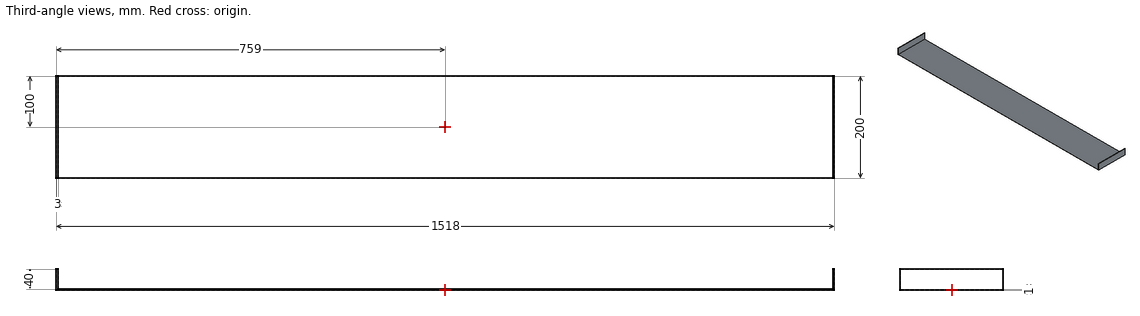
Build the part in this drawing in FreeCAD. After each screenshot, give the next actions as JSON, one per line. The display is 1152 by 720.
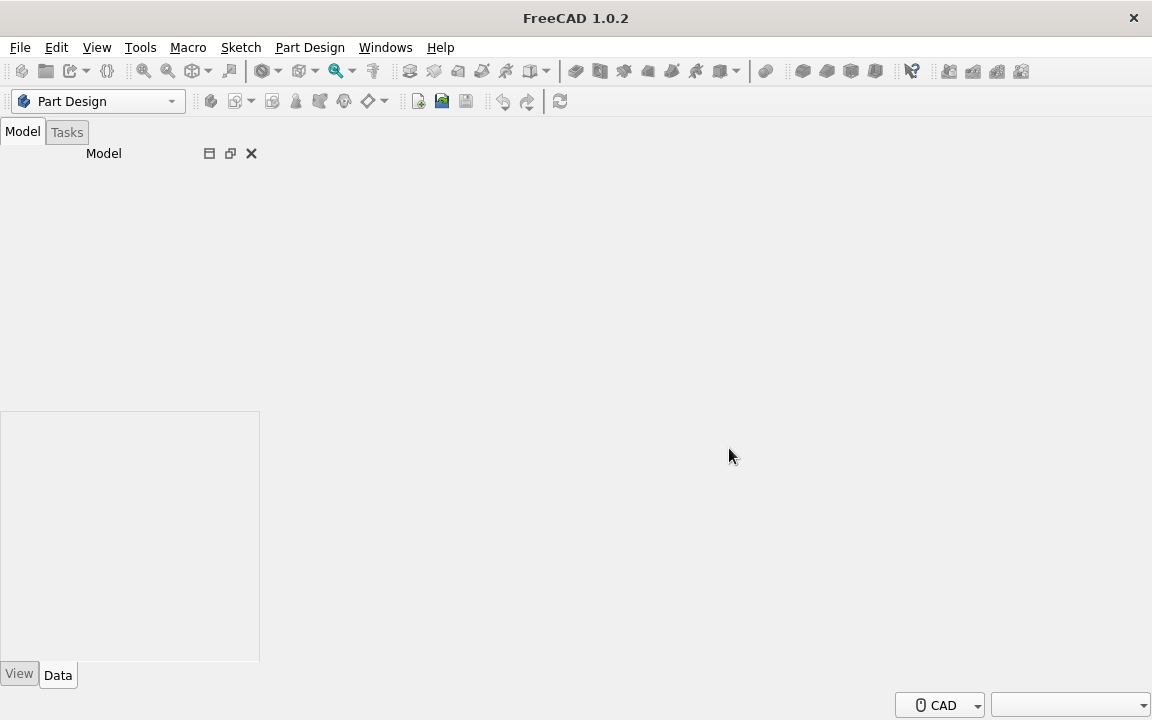
{"action": "left_click", "coordinate": [418, 102]}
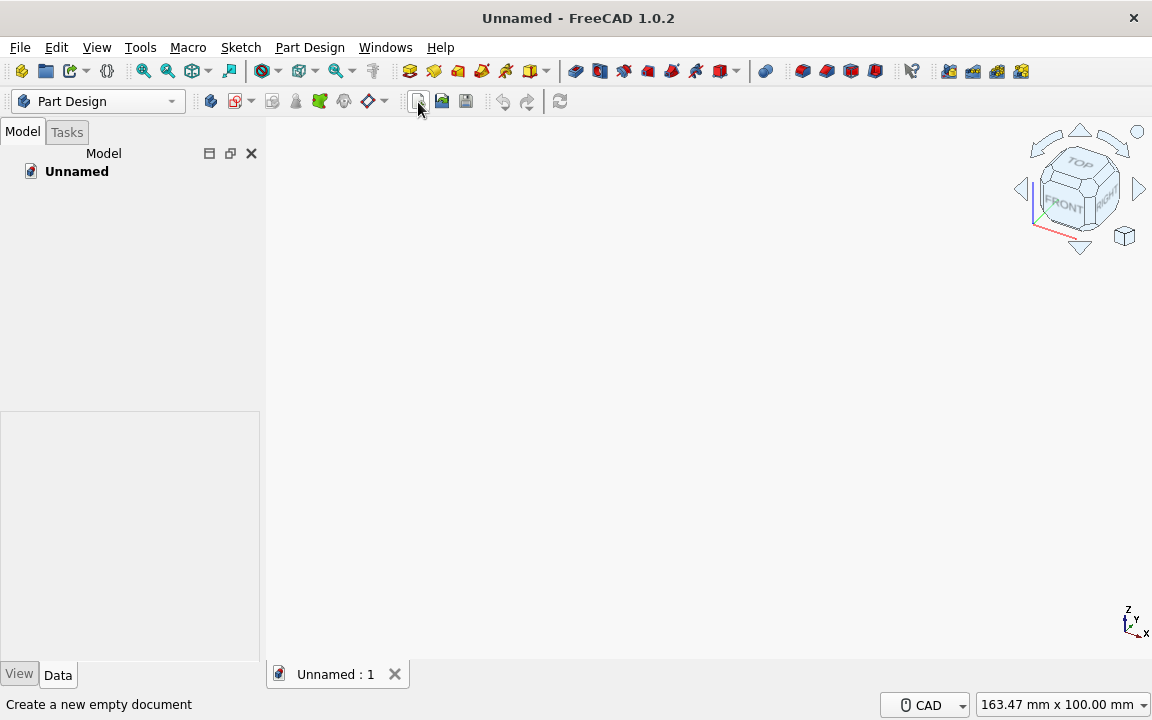
{"action": "left_click", "coordinate": [236, 102]}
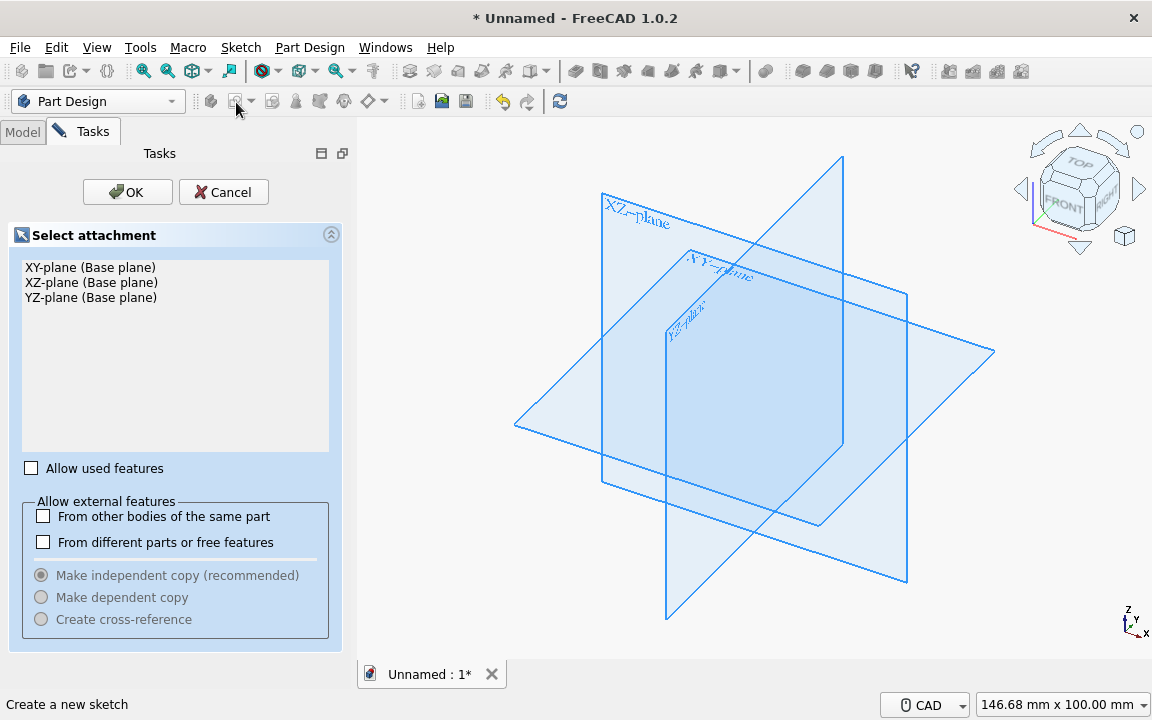
{"action": "left_click", "coordinate": [82, 268]}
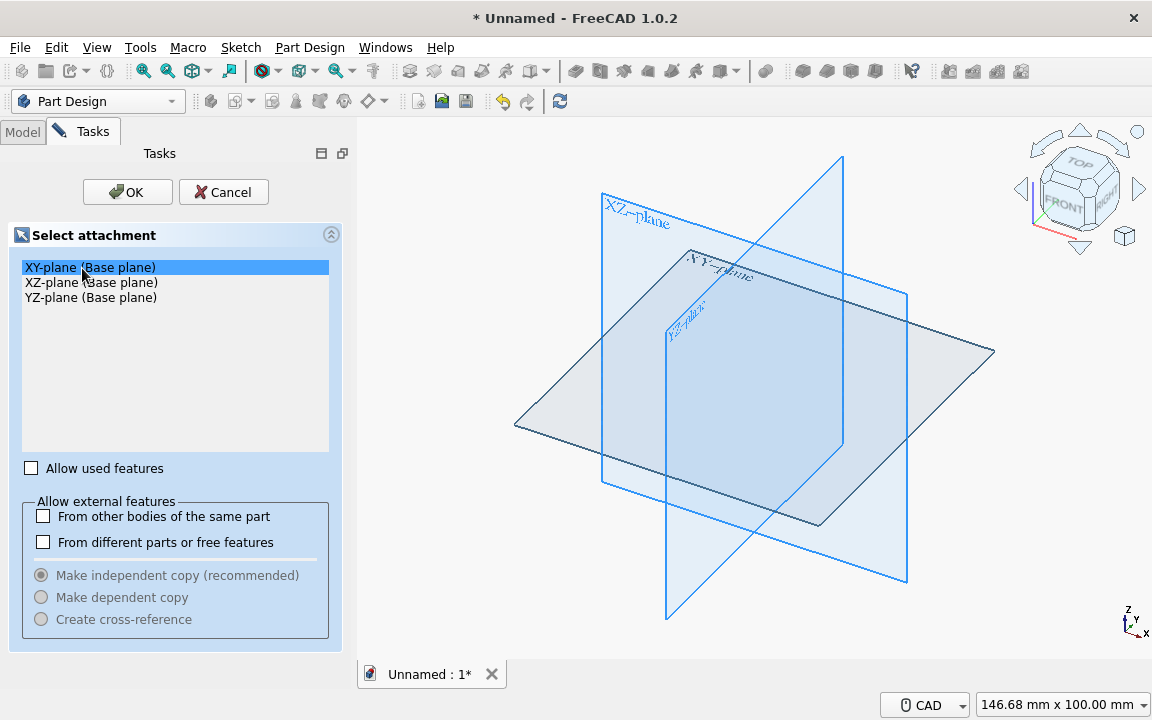
{"action": "left_click", "coordinate": [128, 192]}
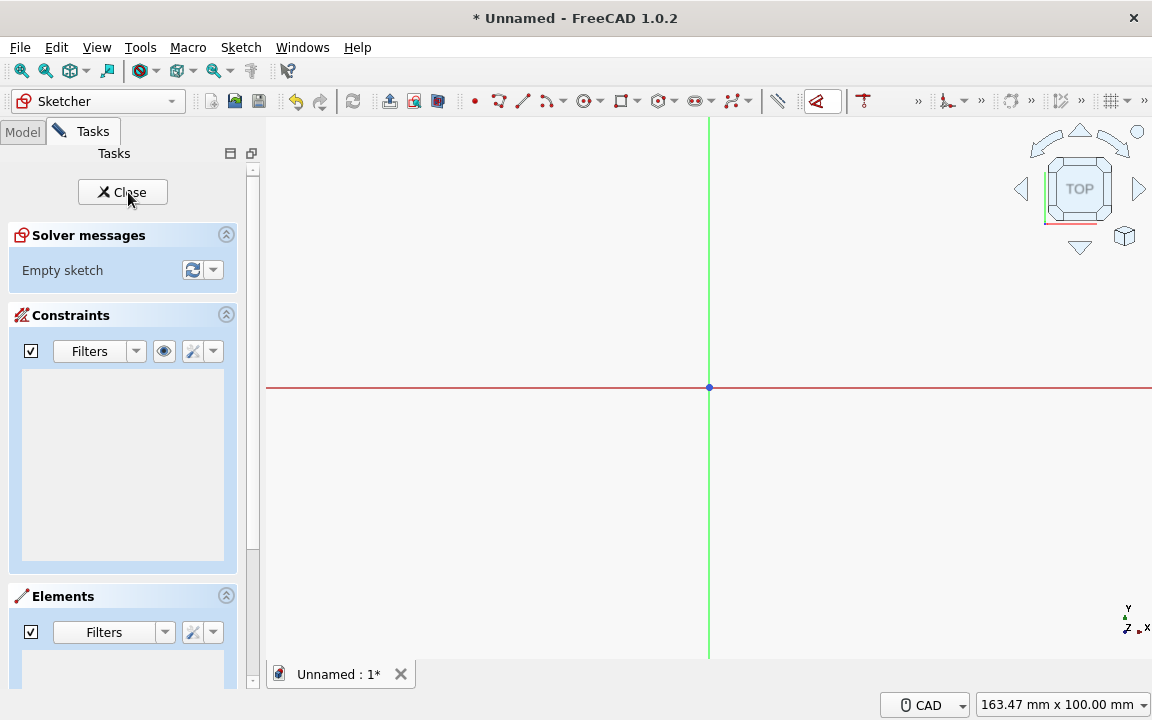
{"action": "scroll", "coordinate": [636, 388], "scroll_direction": "down", "scroll_amount": 14}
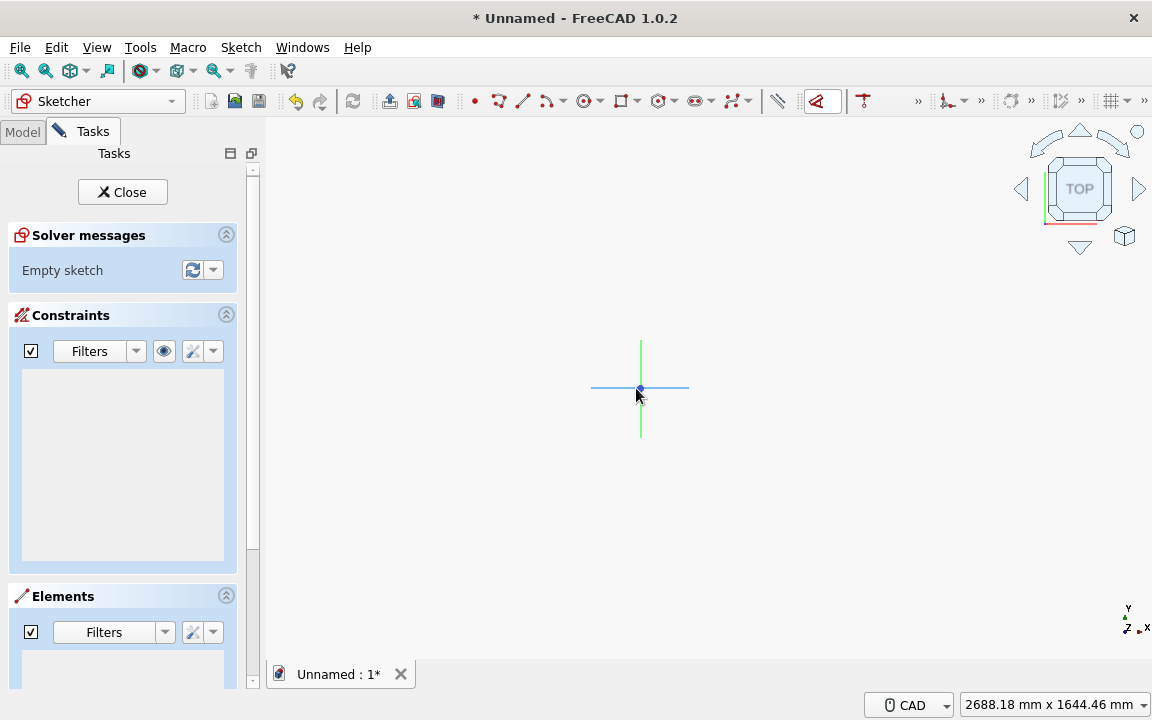
{"action": "left_click", "coordinate": [640, 102]}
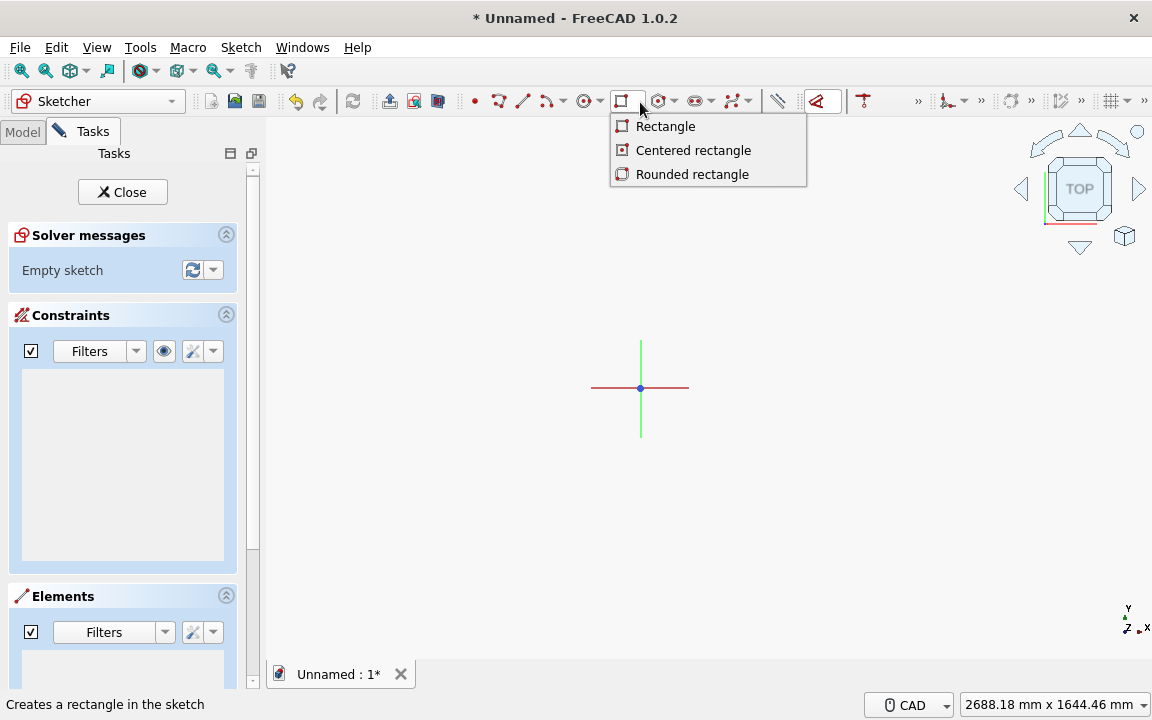
{"action": "left_click", "coordinate": [708, 150]}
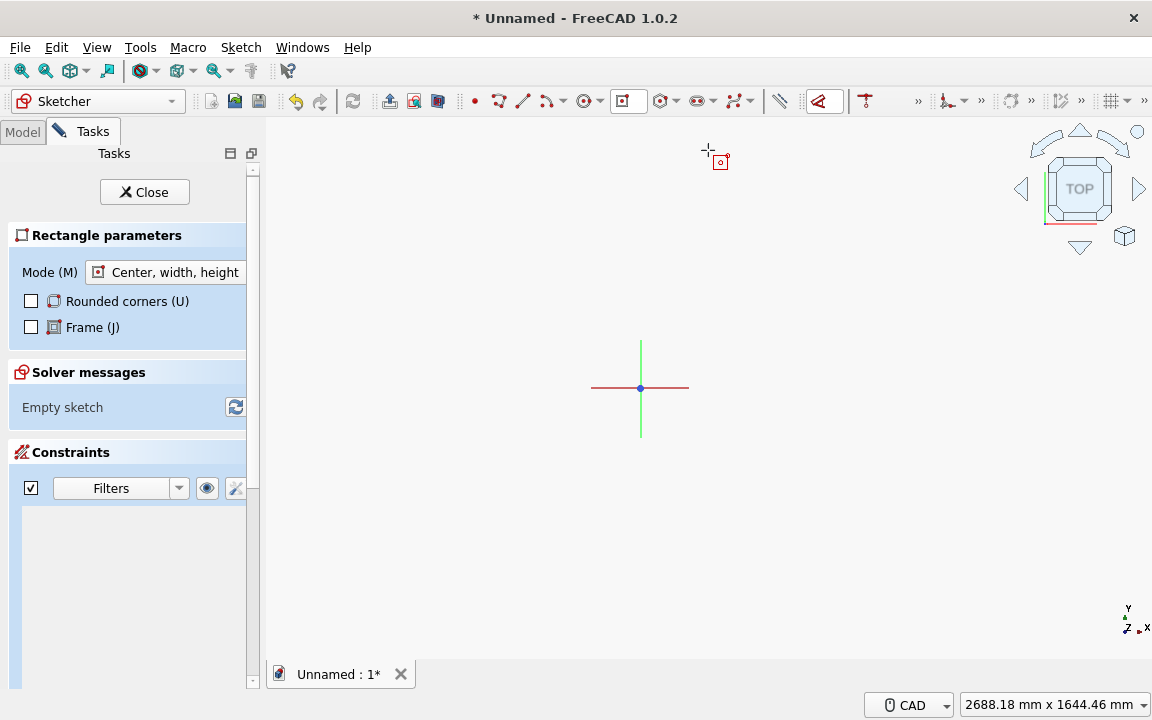
{"action": "left_click", "coordinate": [641, 388]}
{"action": "mouse_move", "coordinate": [891, 356]}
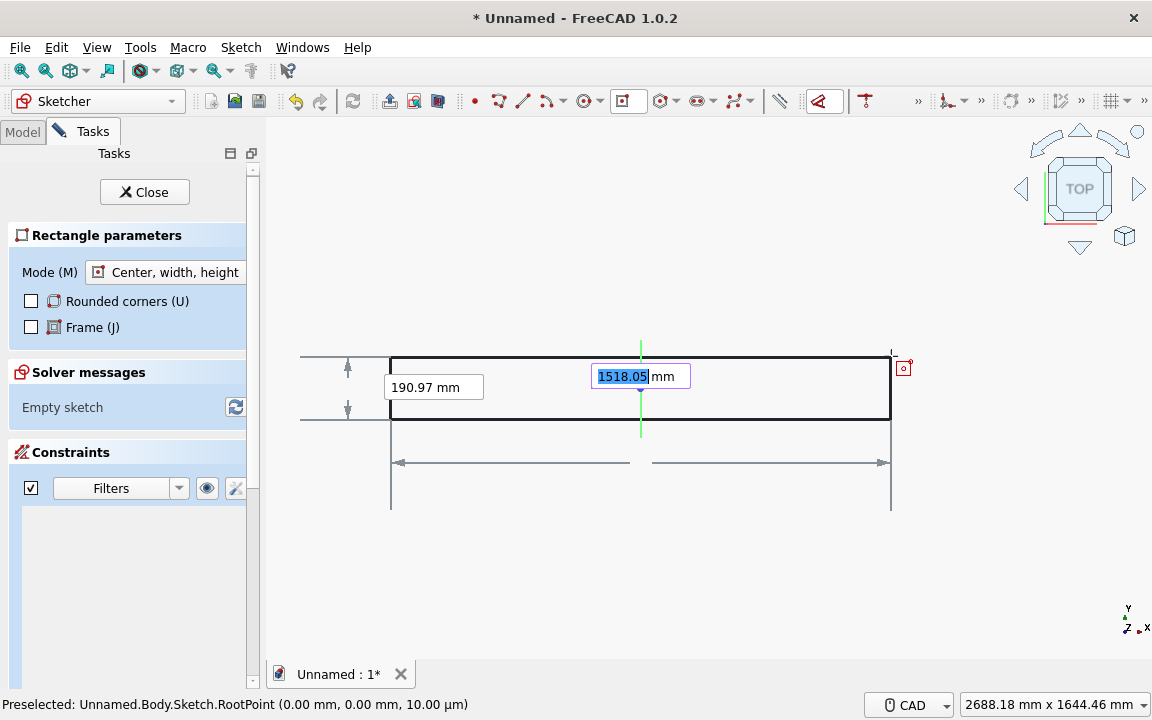
{"action": "type", "text": "1518"}
{"action": "key", "text": "Tab"}
{"action": "type", "text": "200"}
{"action": "key", "text": "Return"}
{"action": "key", "text": "Escape"}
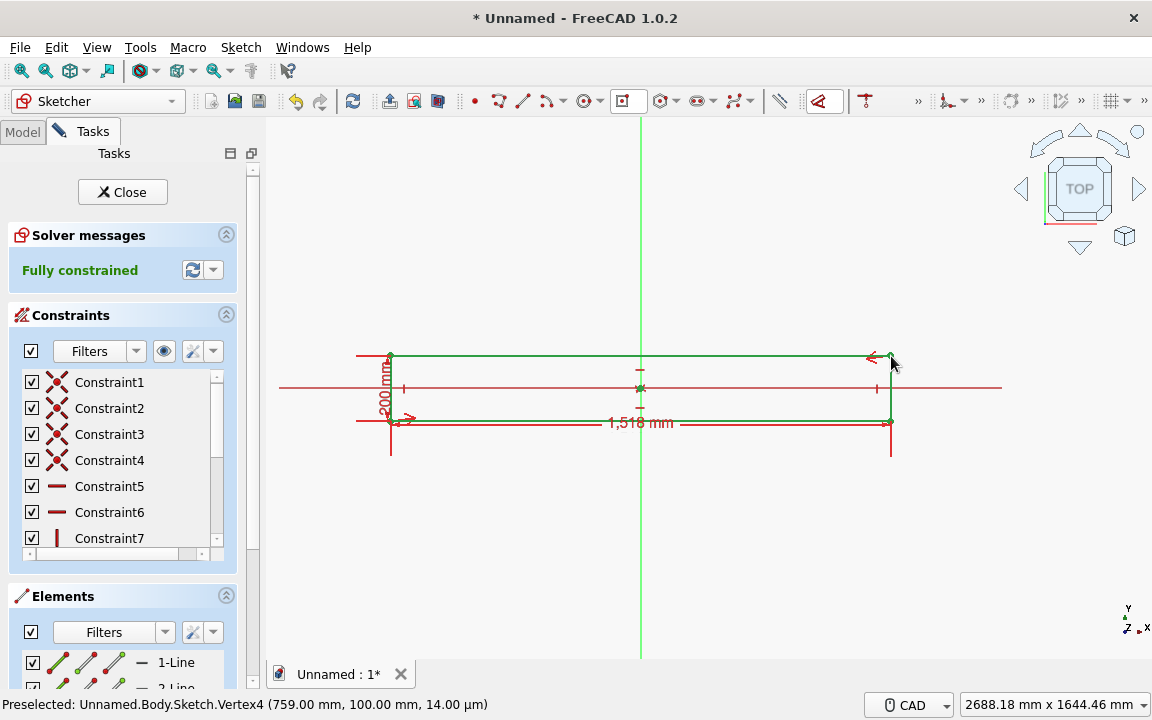
{"action": "left_click", "coordinate": [123, 192]}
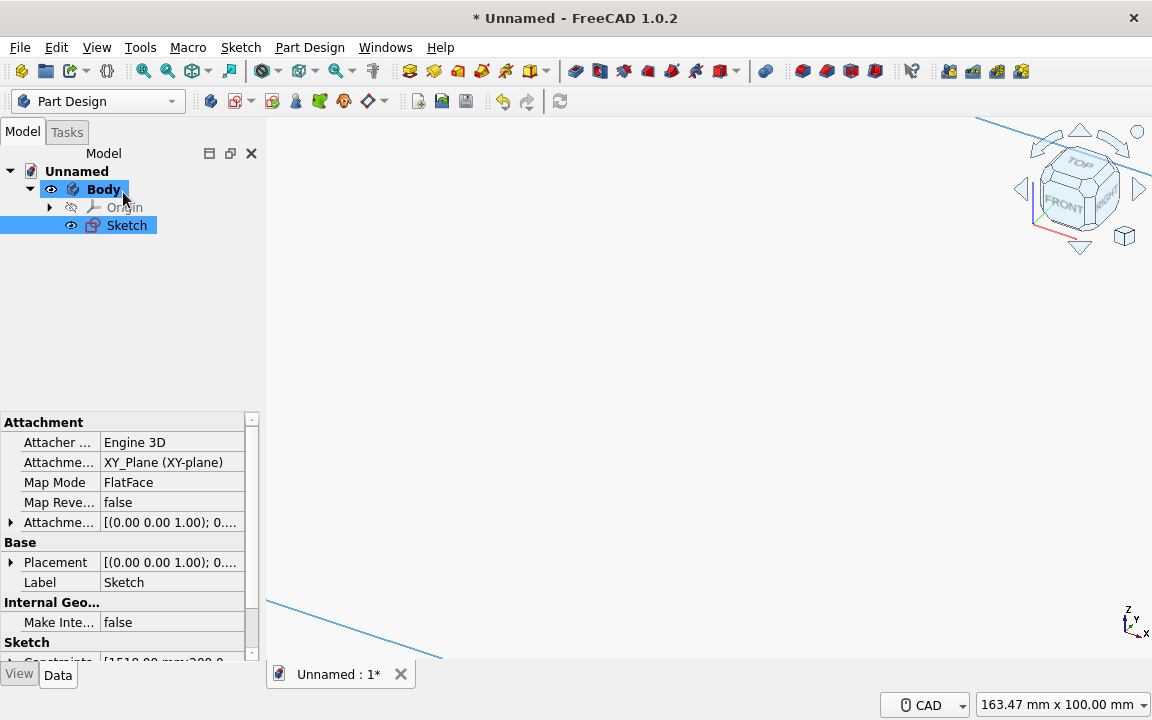
{"action": "left_click", "coordinate": [410, 72]}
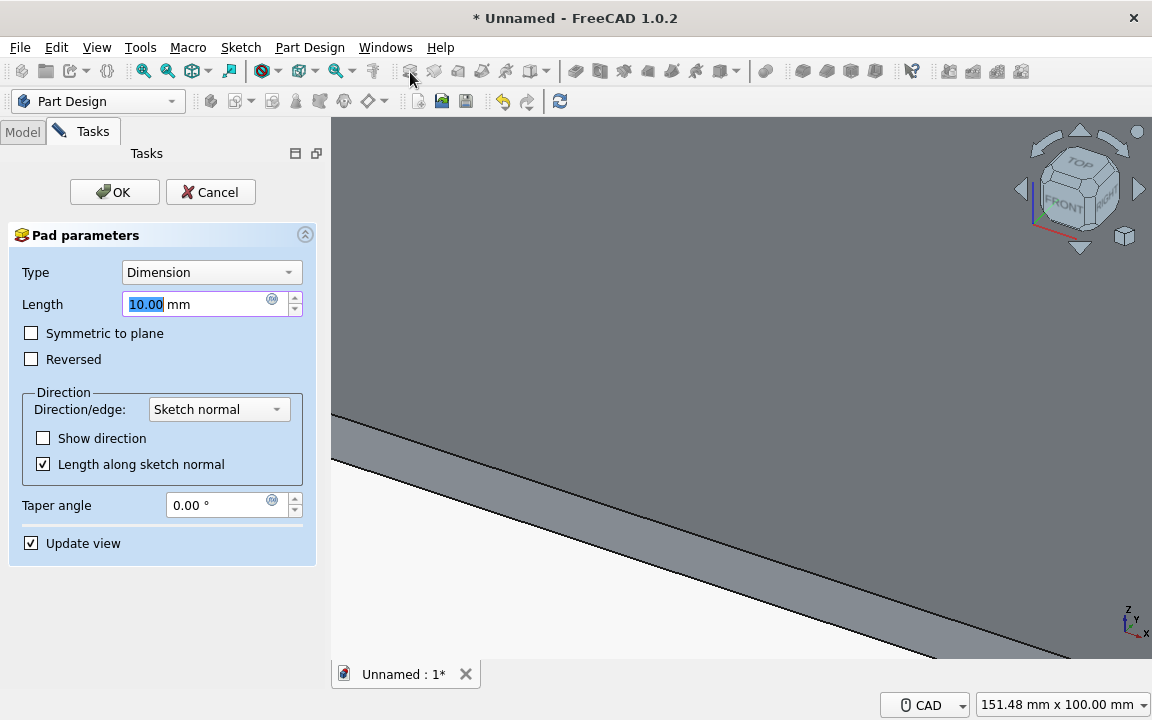
{"action": "type", "text": "1"}
{"action": "key", "text": "Tab"}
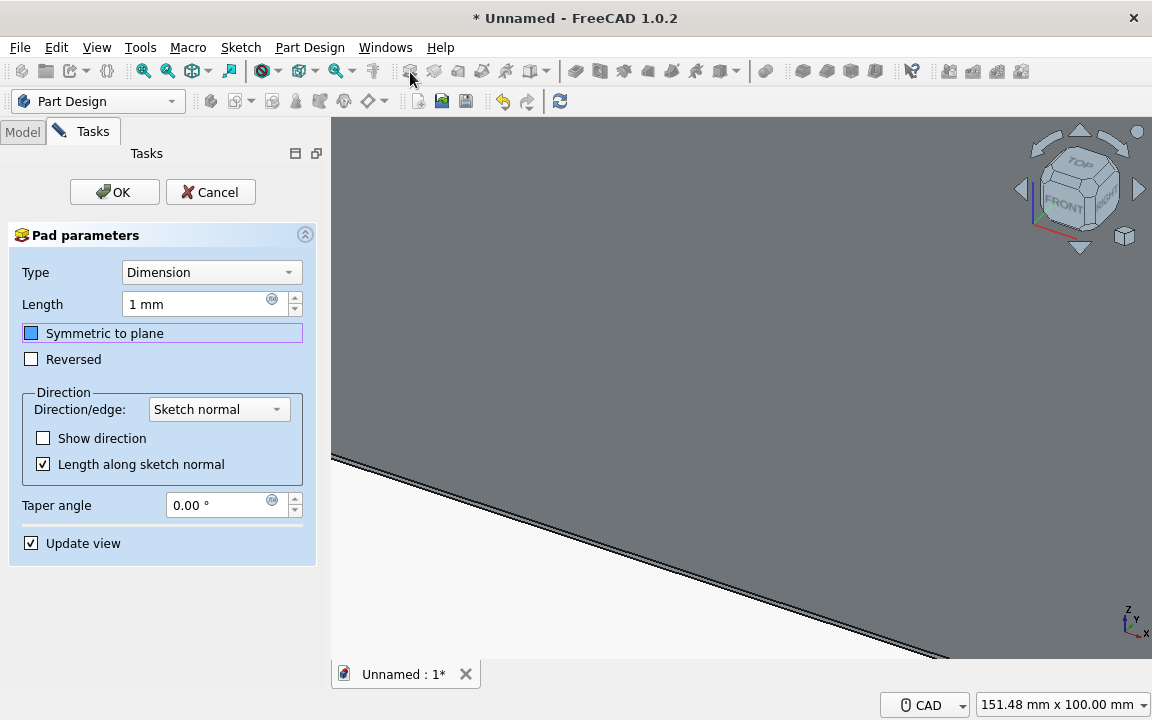
{"action": "left_click", "coordinate": [115, 192]}